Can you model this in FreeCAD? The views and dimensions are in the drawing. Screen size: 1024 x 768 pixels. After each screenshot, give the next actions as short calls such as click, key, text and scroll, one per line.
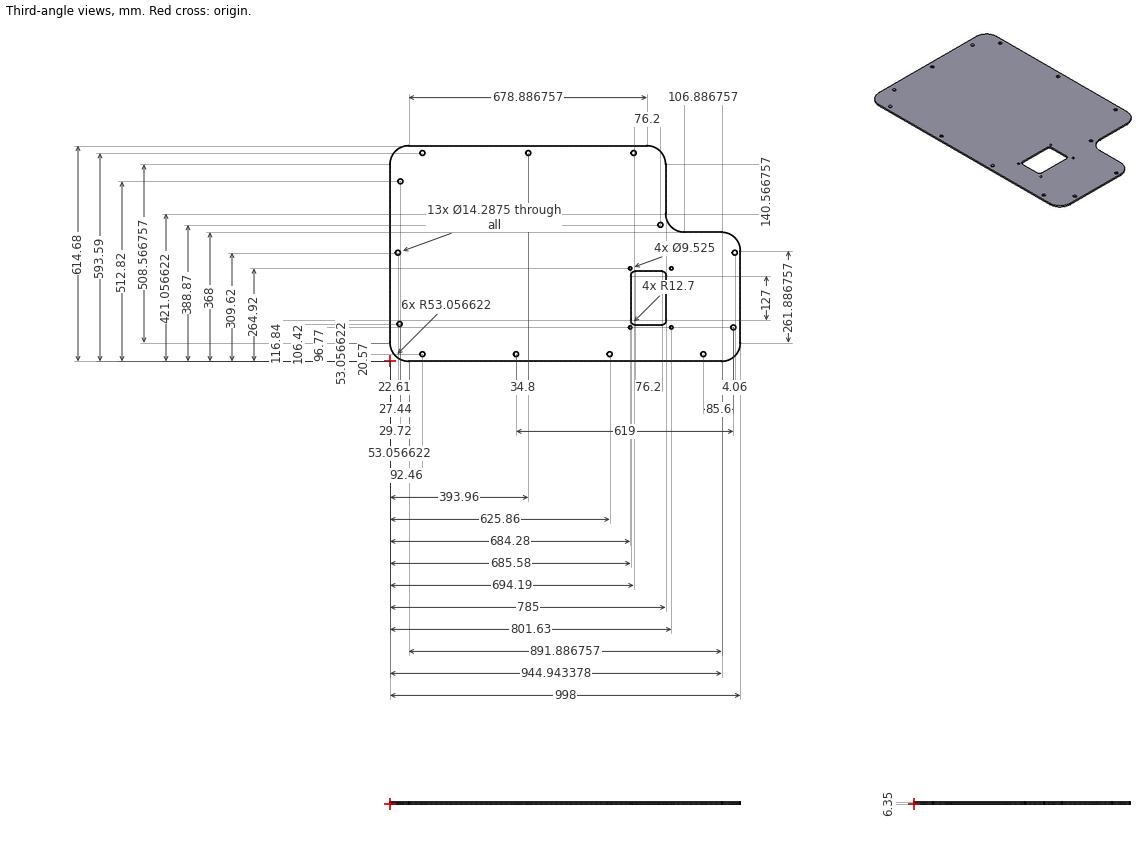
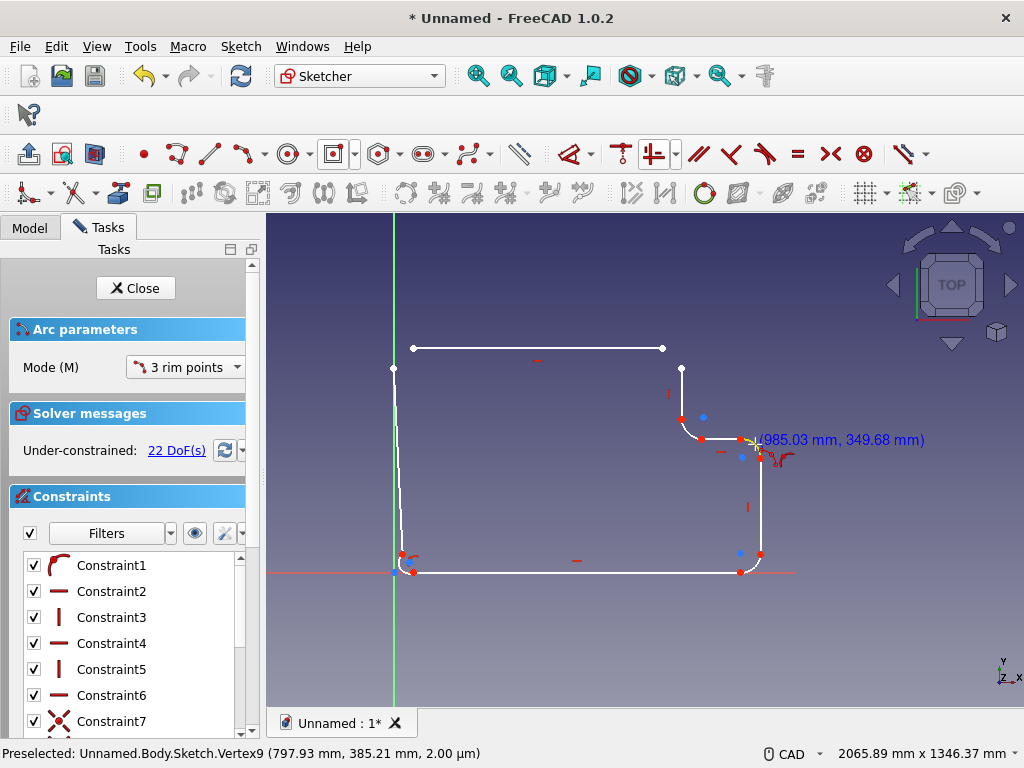
click(682, 368)
click(663, 348)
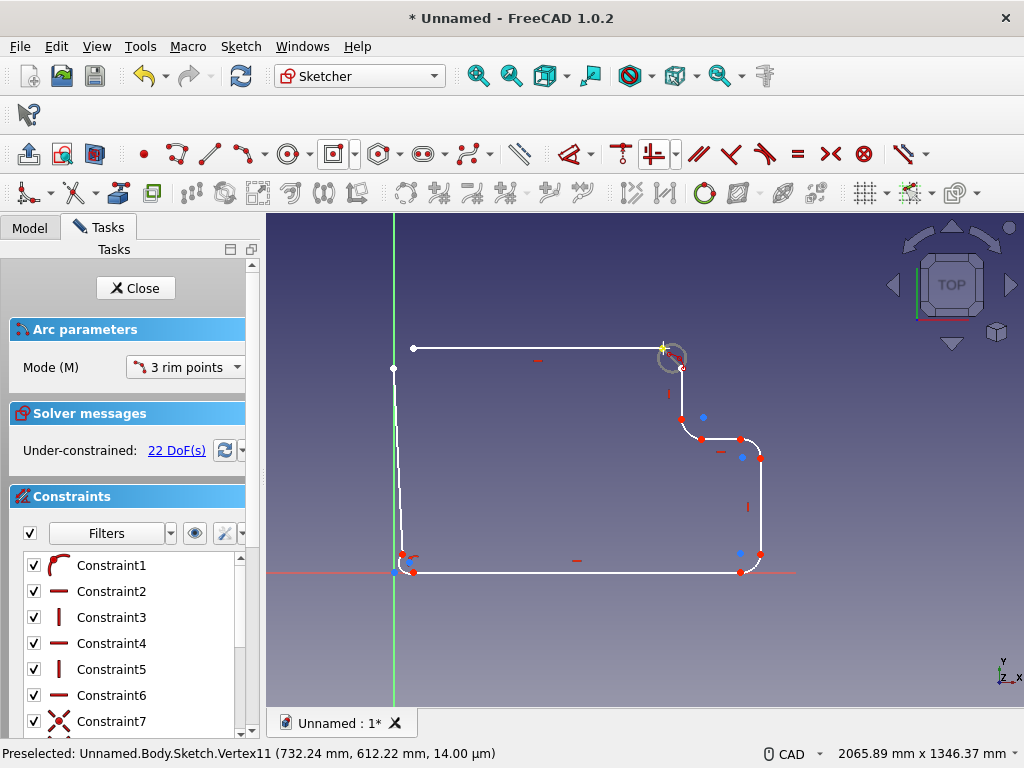
scroll(676, 353, up, 6)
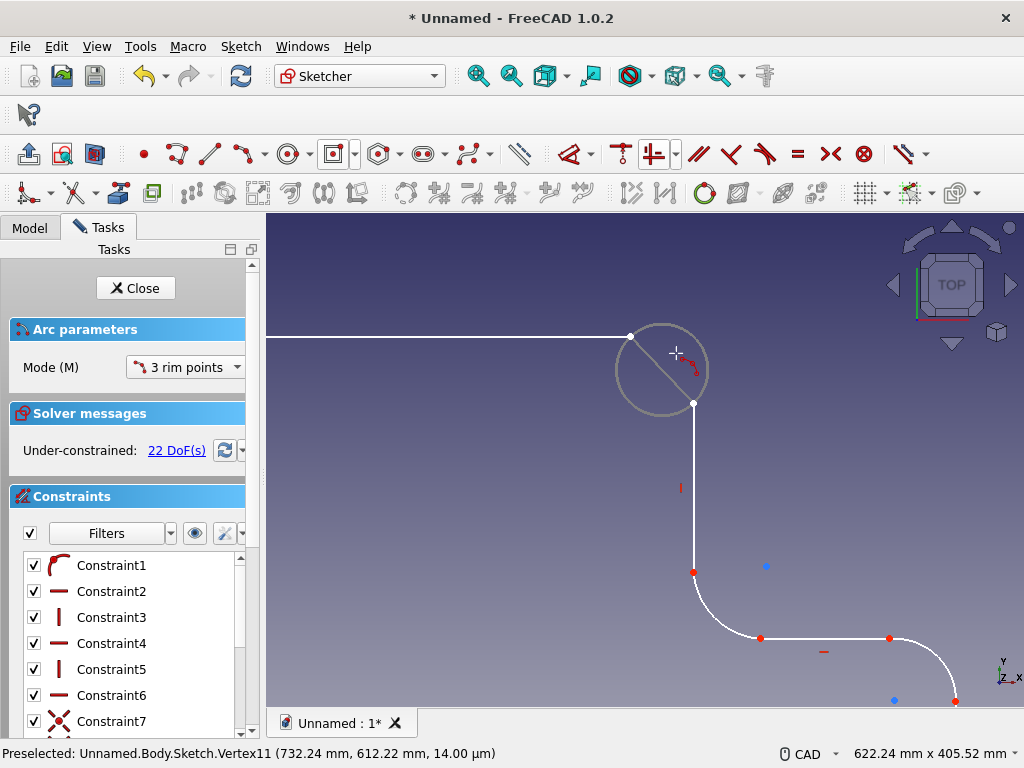
click(676, 353)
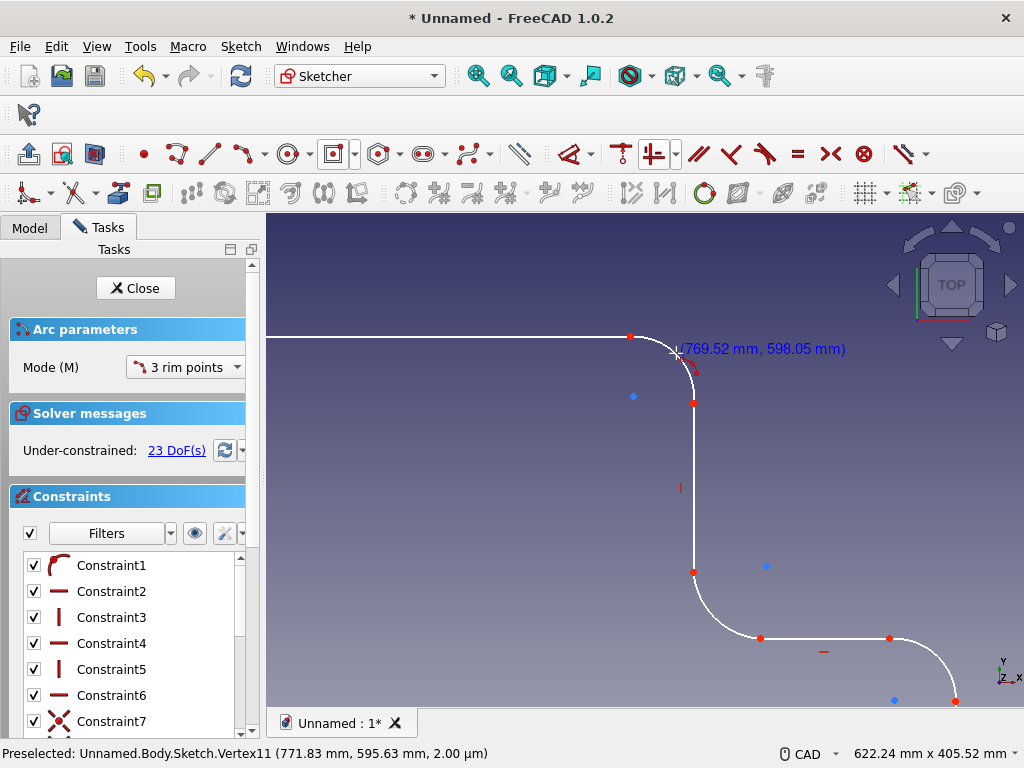
scroll(676, 353, down, 6)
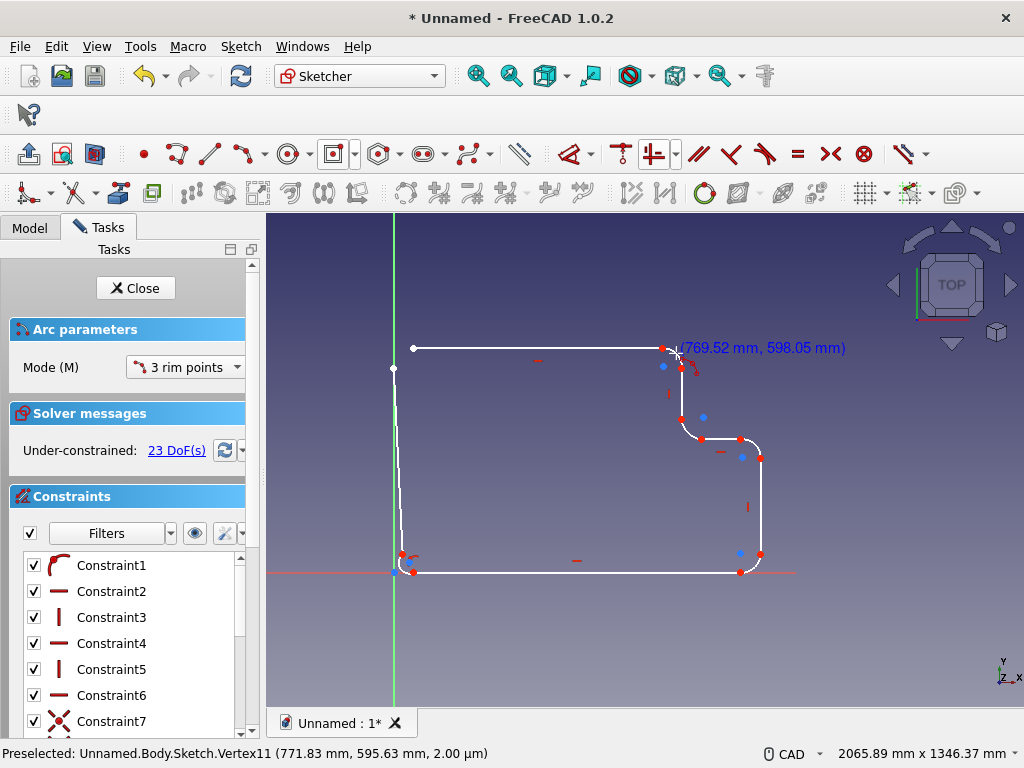
click(414, 348)
click(394, 368)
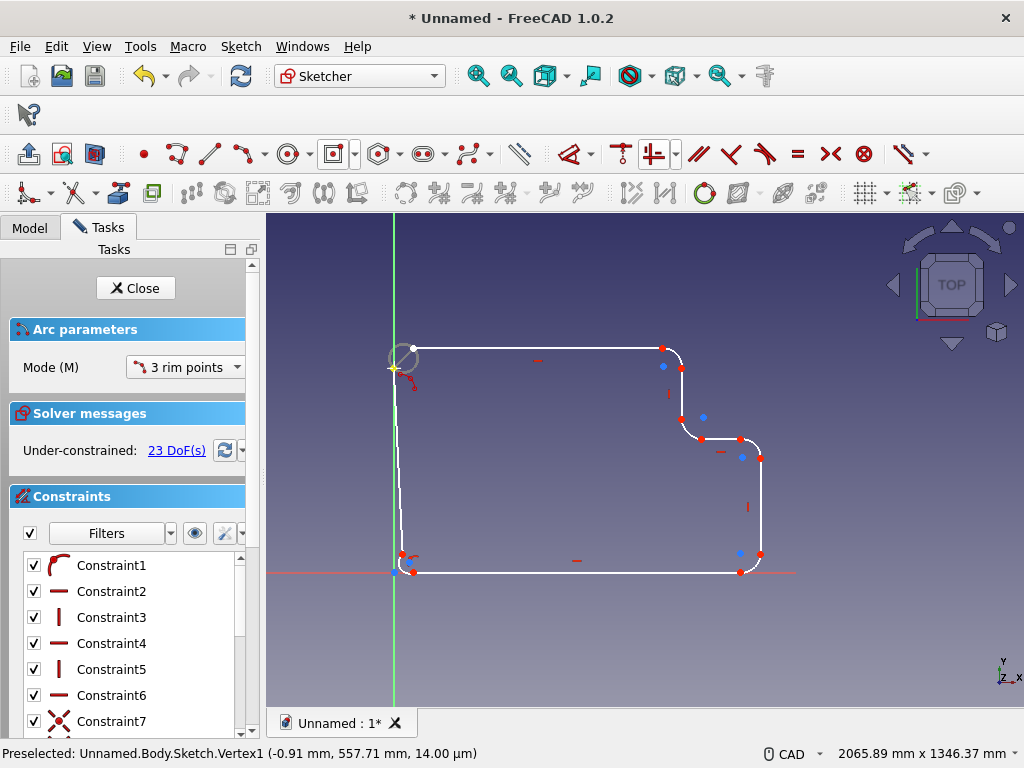
scroll(400, 353, up, 6)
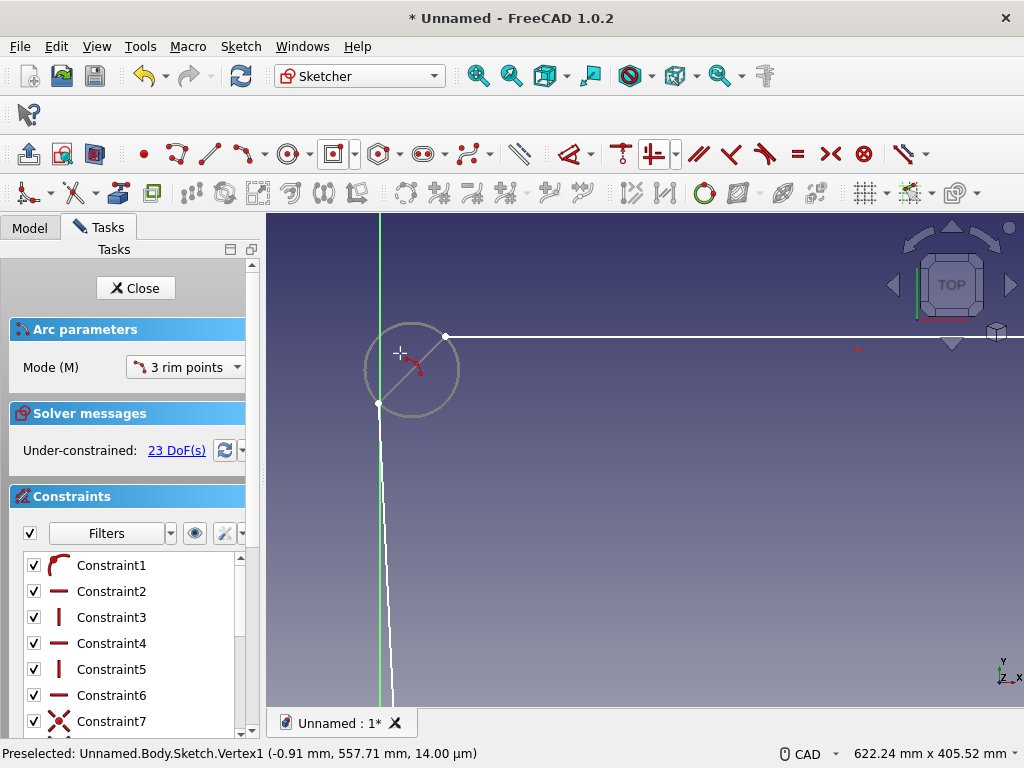
click(399, 353)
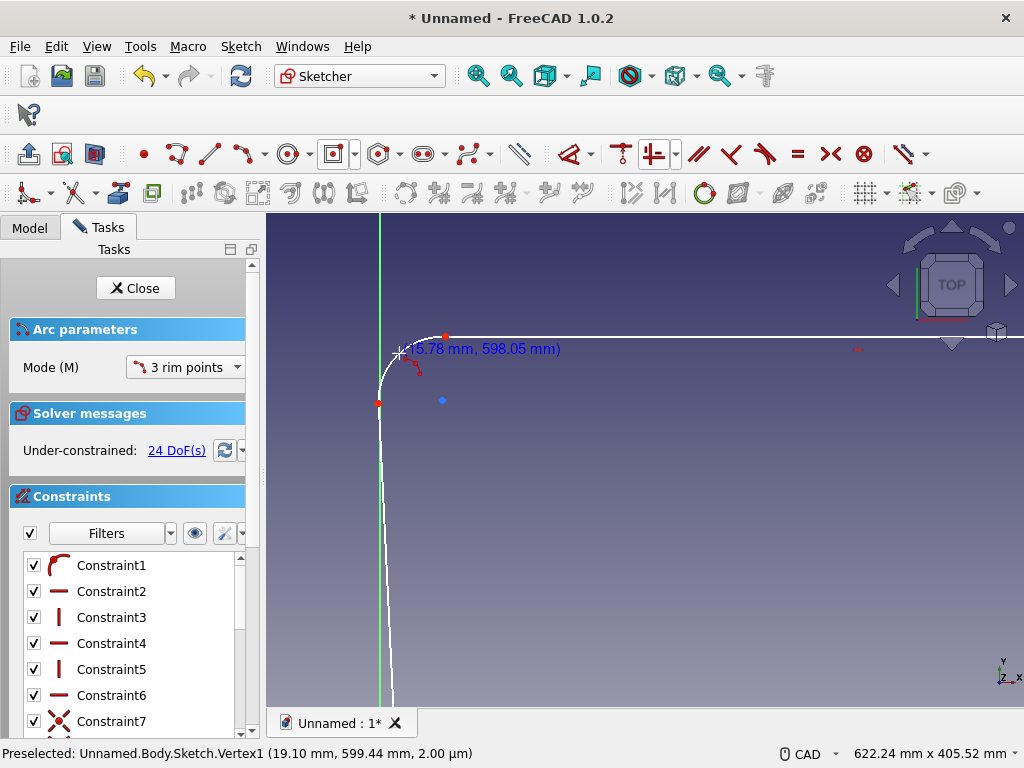
click(210, 154)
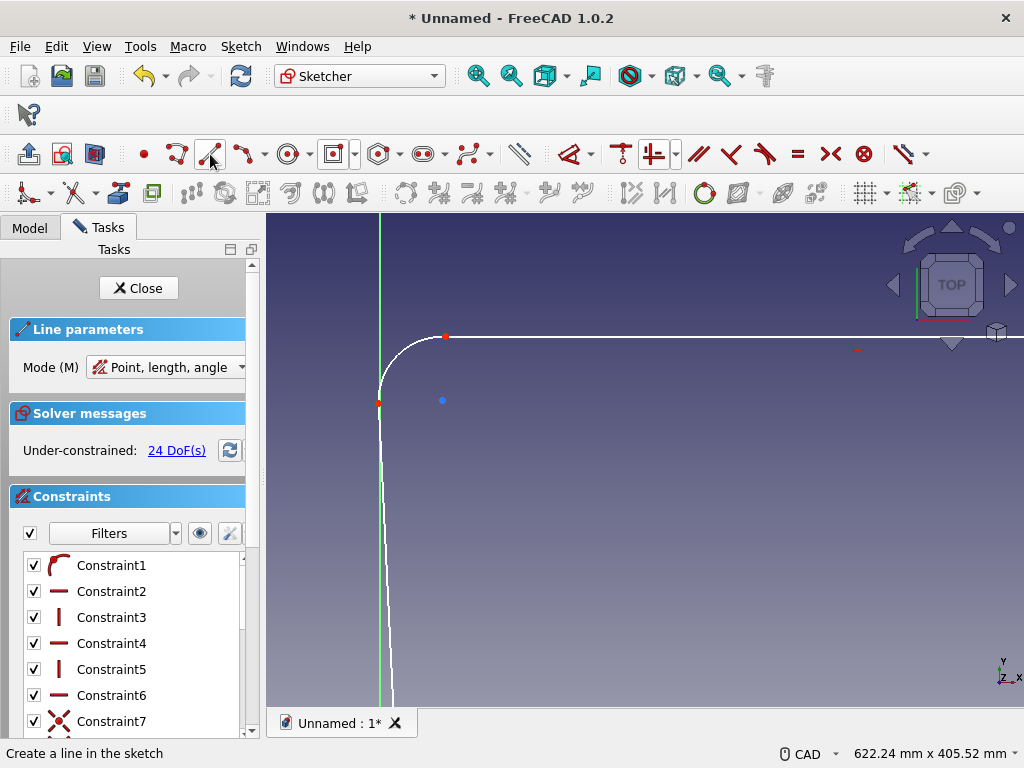
scroll(399, 353, down, 6)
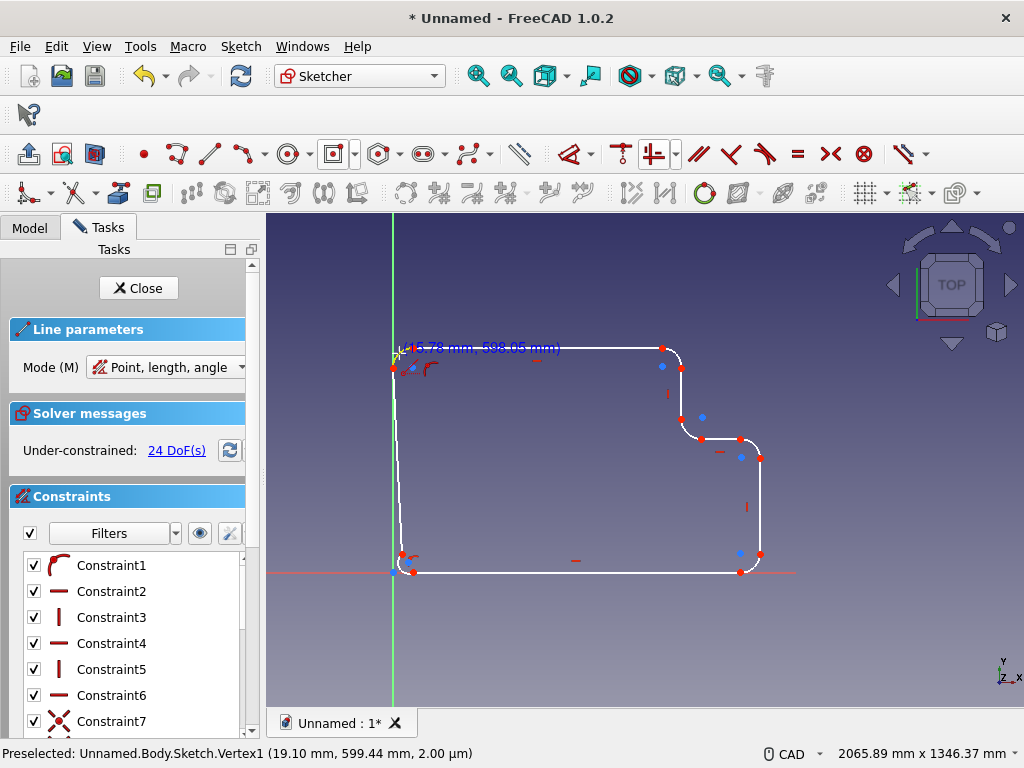
click(645, 530)
click(645, 483)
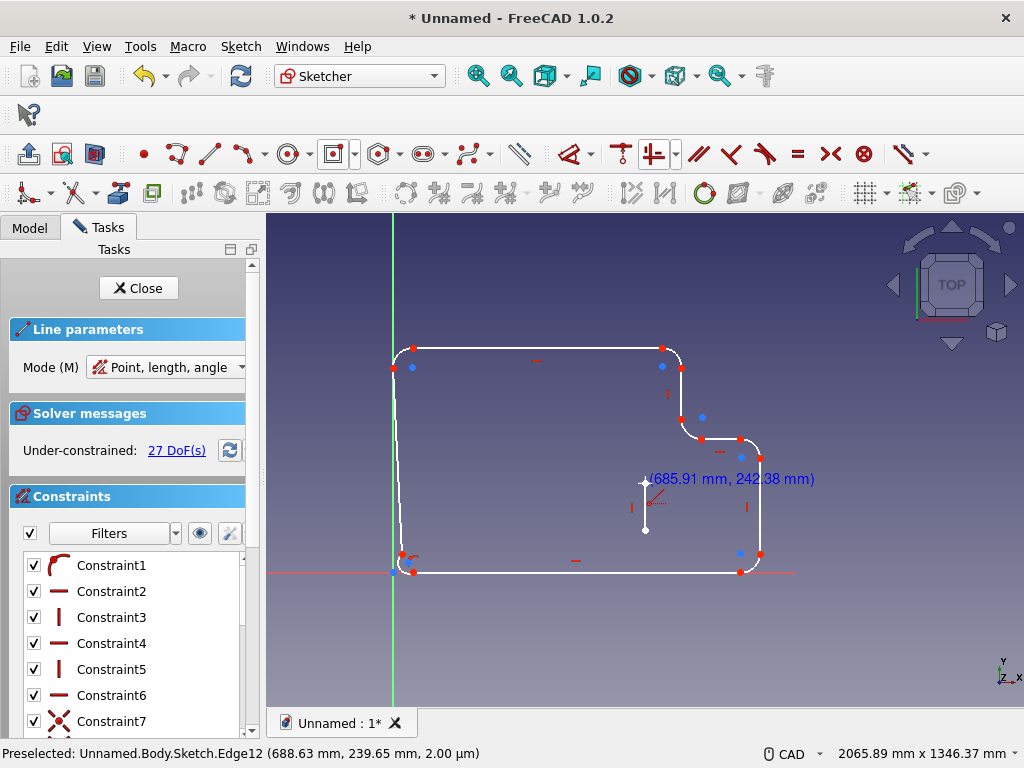
scroll(650, 479, up, 5)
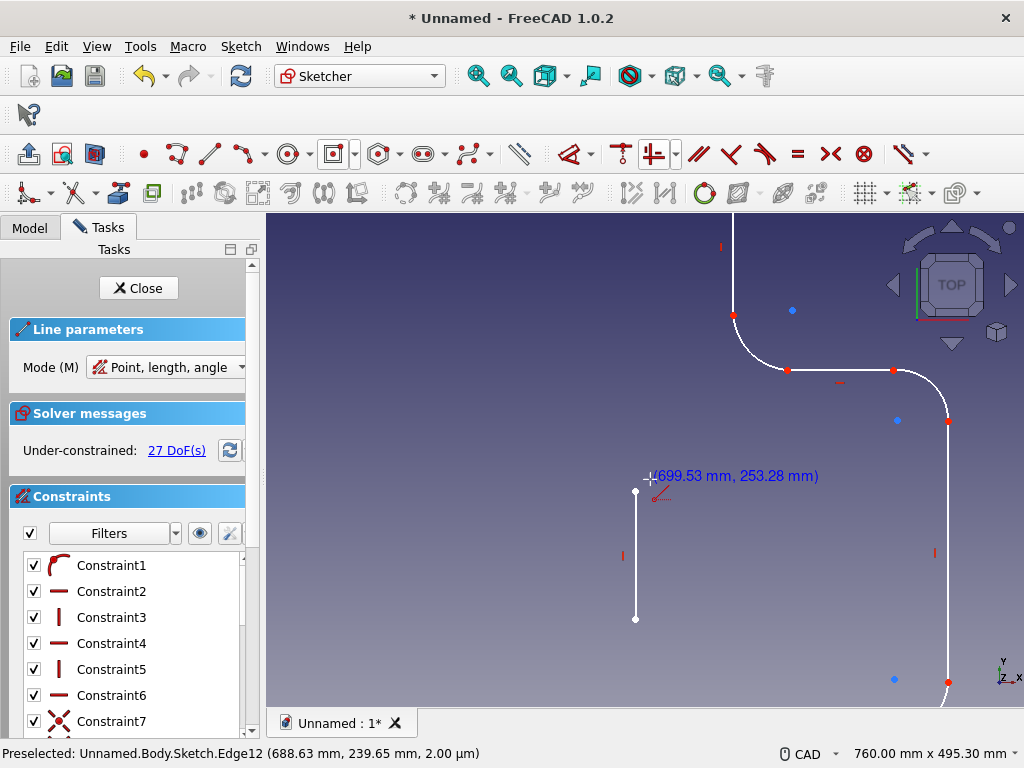
click(648, 478)
click(724, 478)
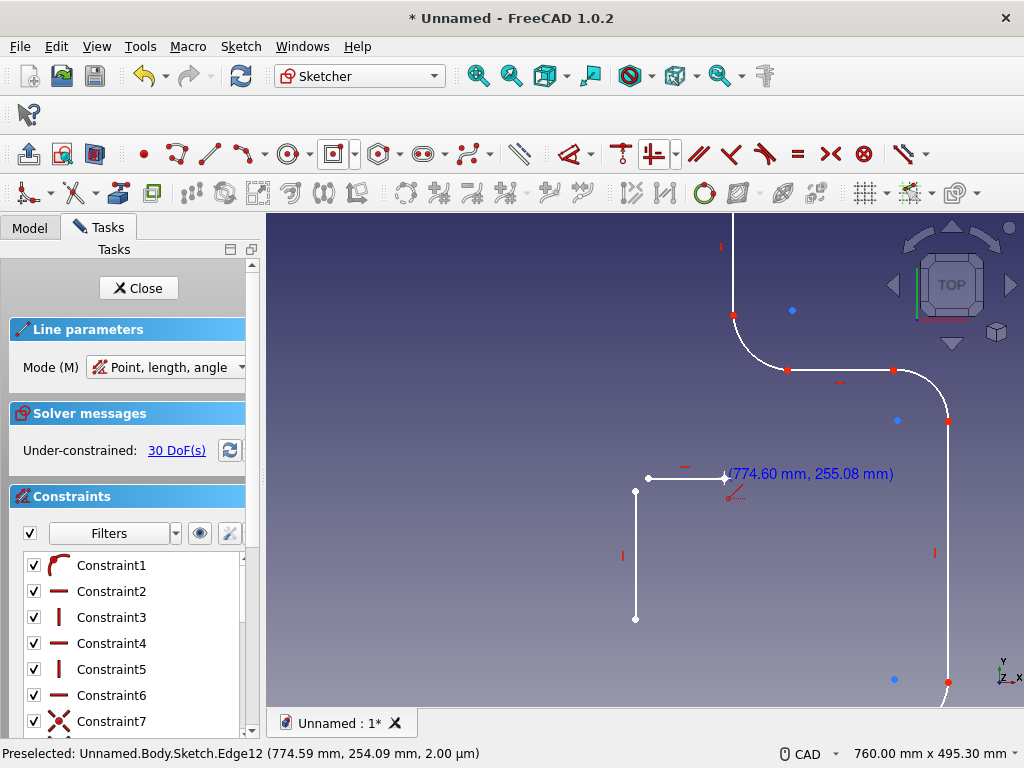
click(737, 490)
click(737, 617)